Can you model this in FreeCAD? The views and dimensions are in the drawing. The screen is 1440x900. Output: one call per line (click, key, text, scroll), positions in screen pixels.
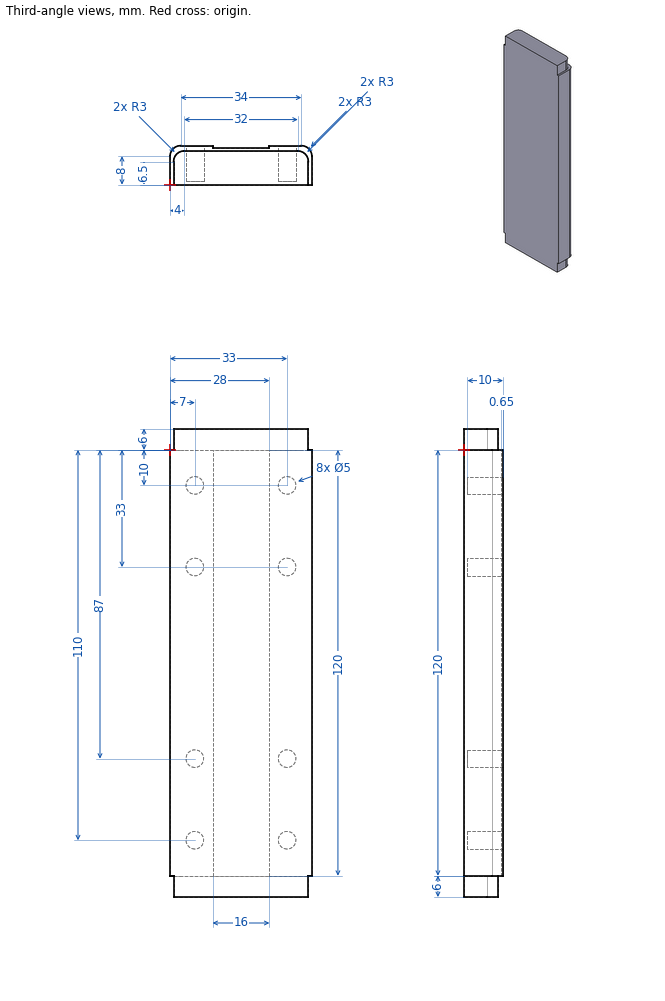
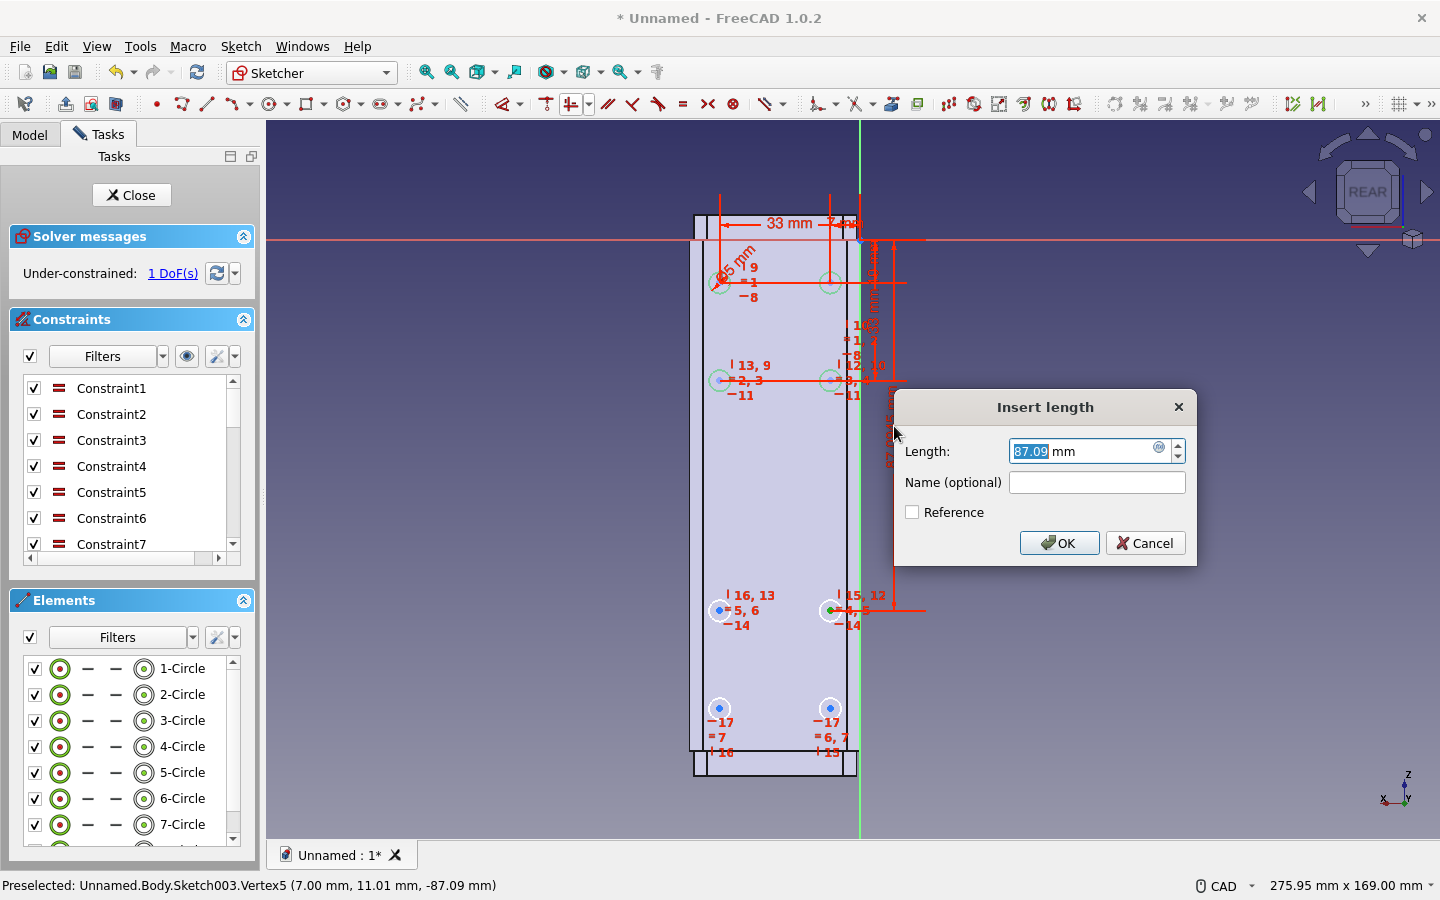
text(87)
key(Return)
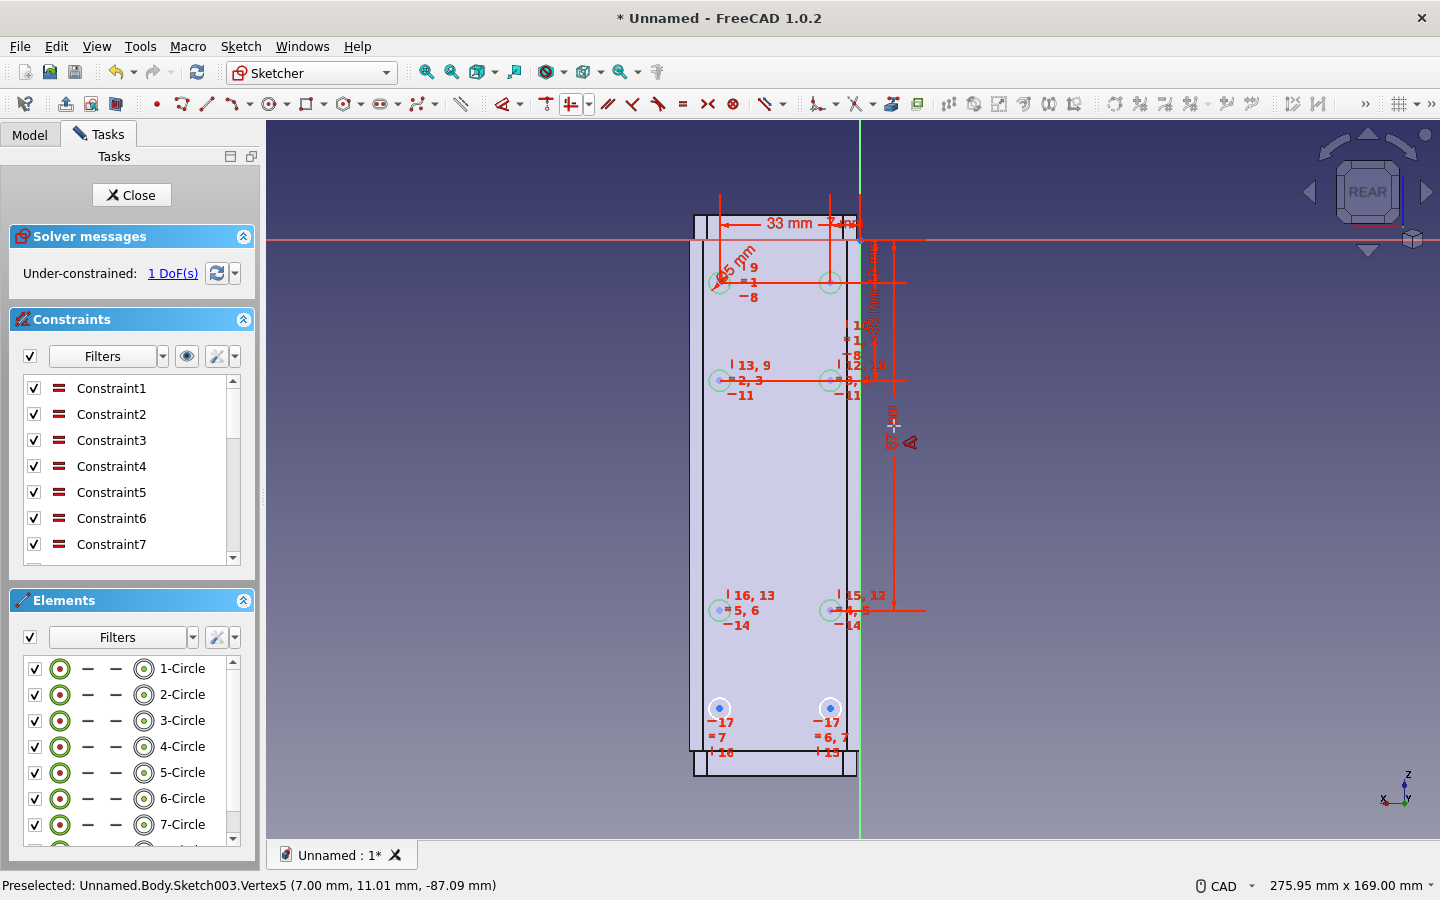
click(830, 709)
click(894, 475)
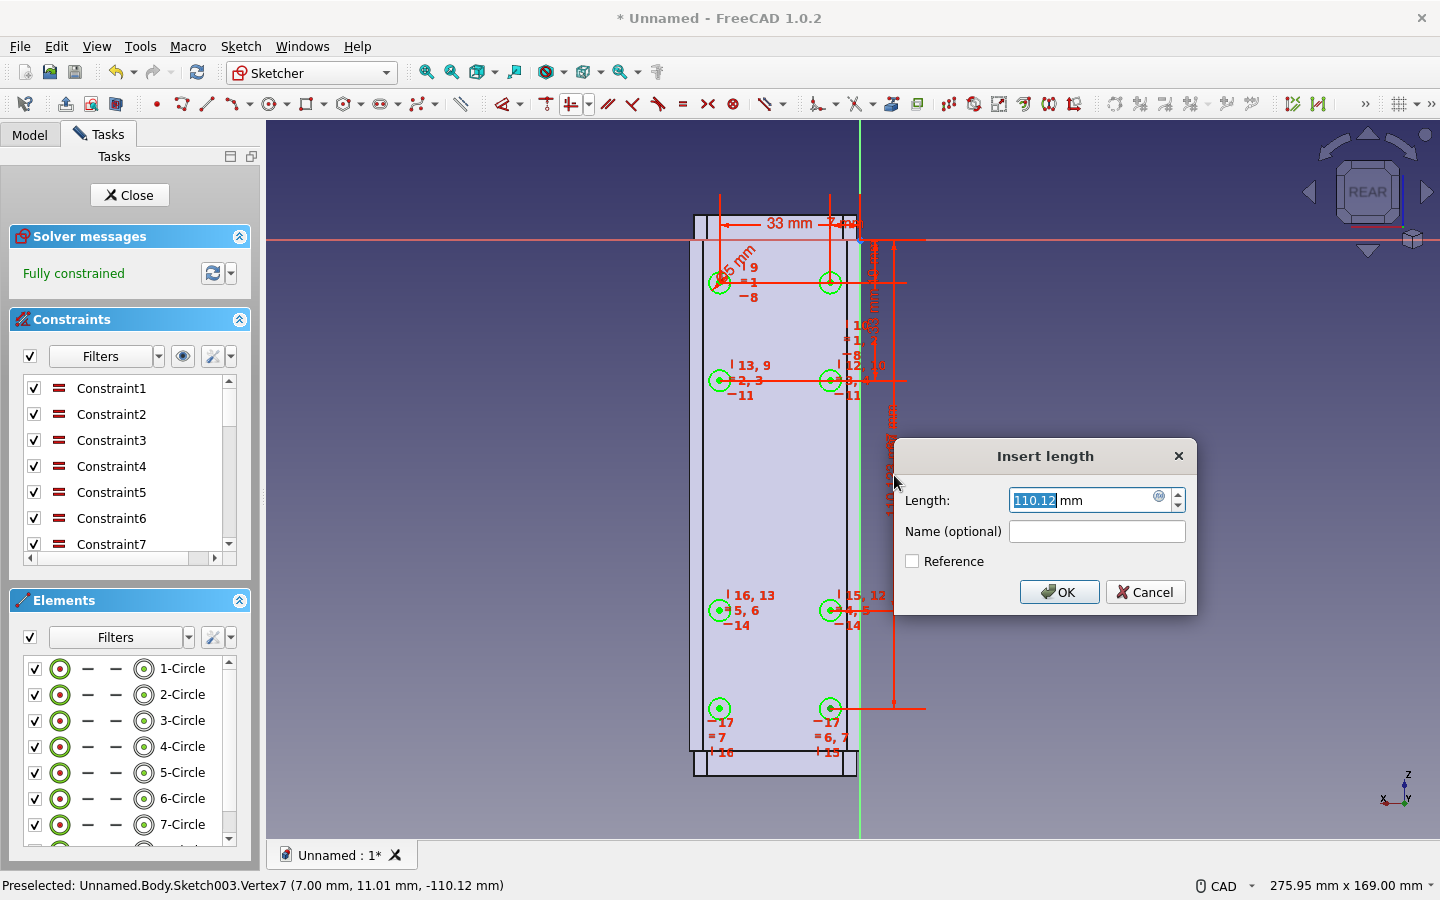
text(110)
key(Return)
key(Escape)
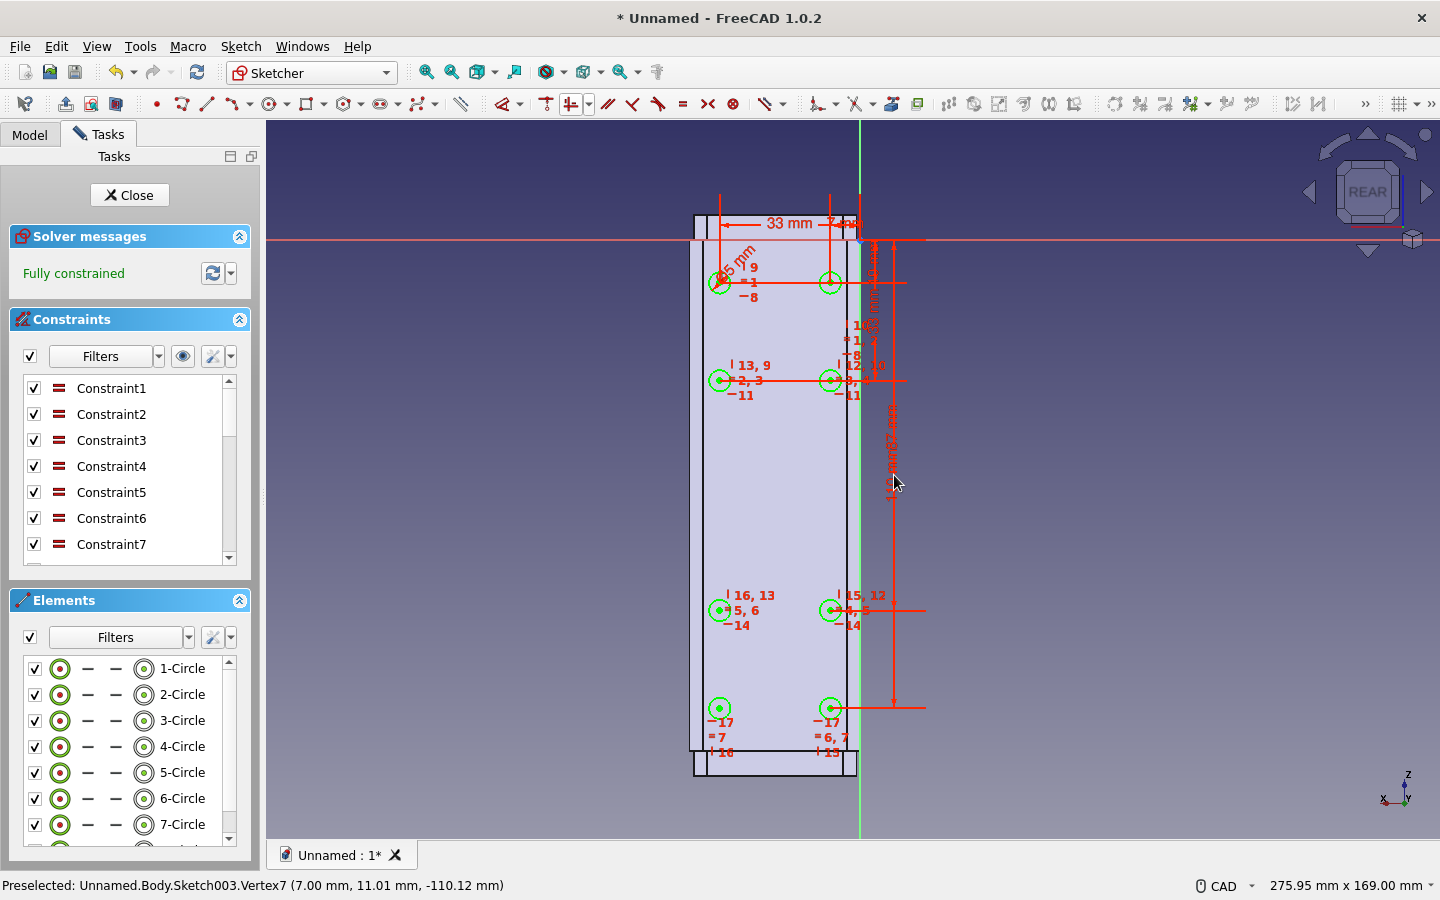
click(130, 195)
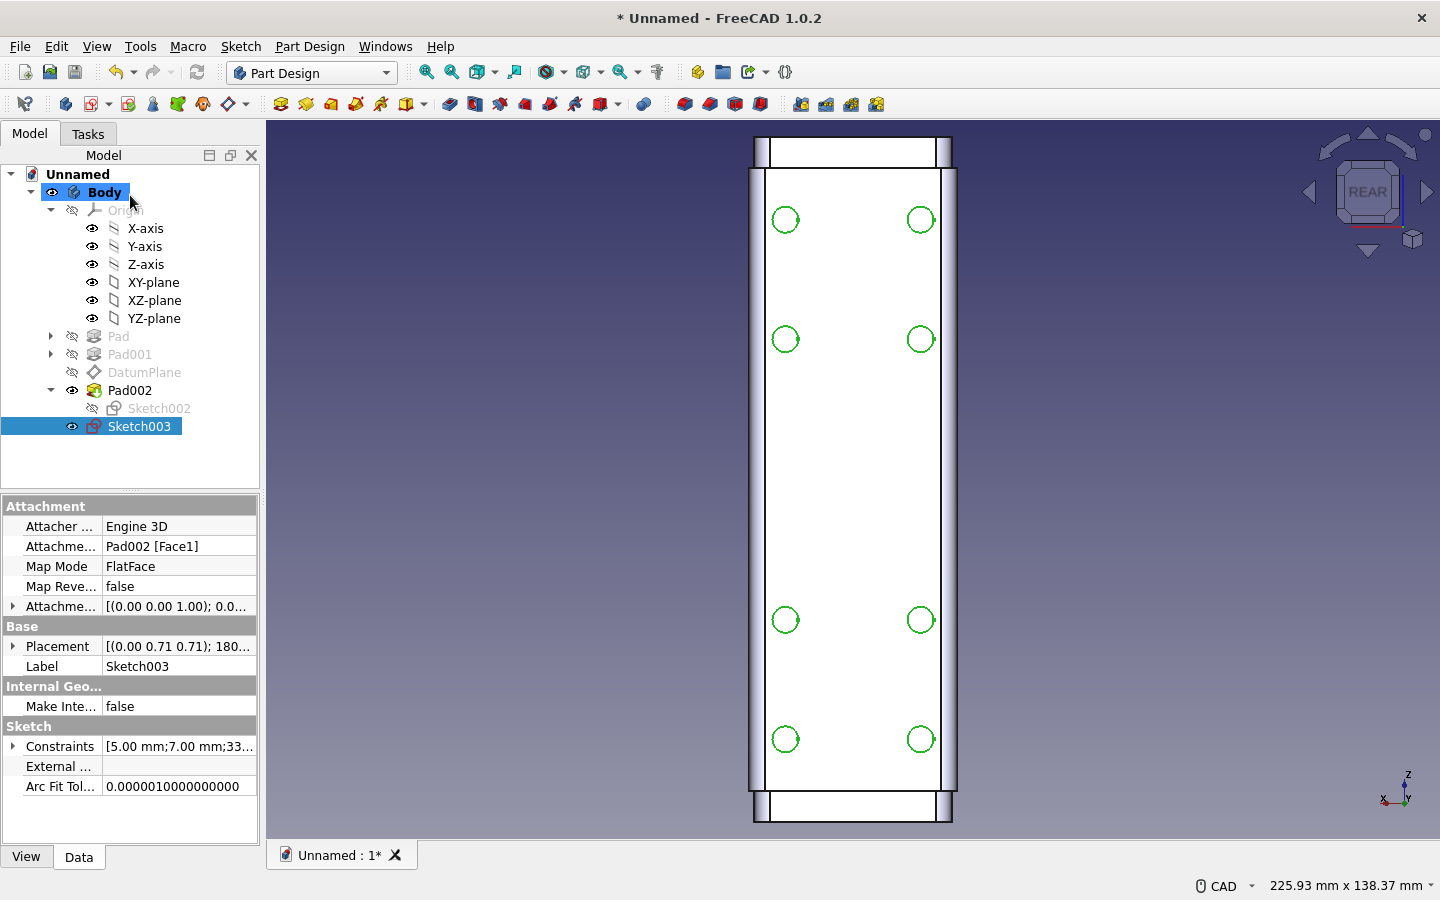
click(450, 104)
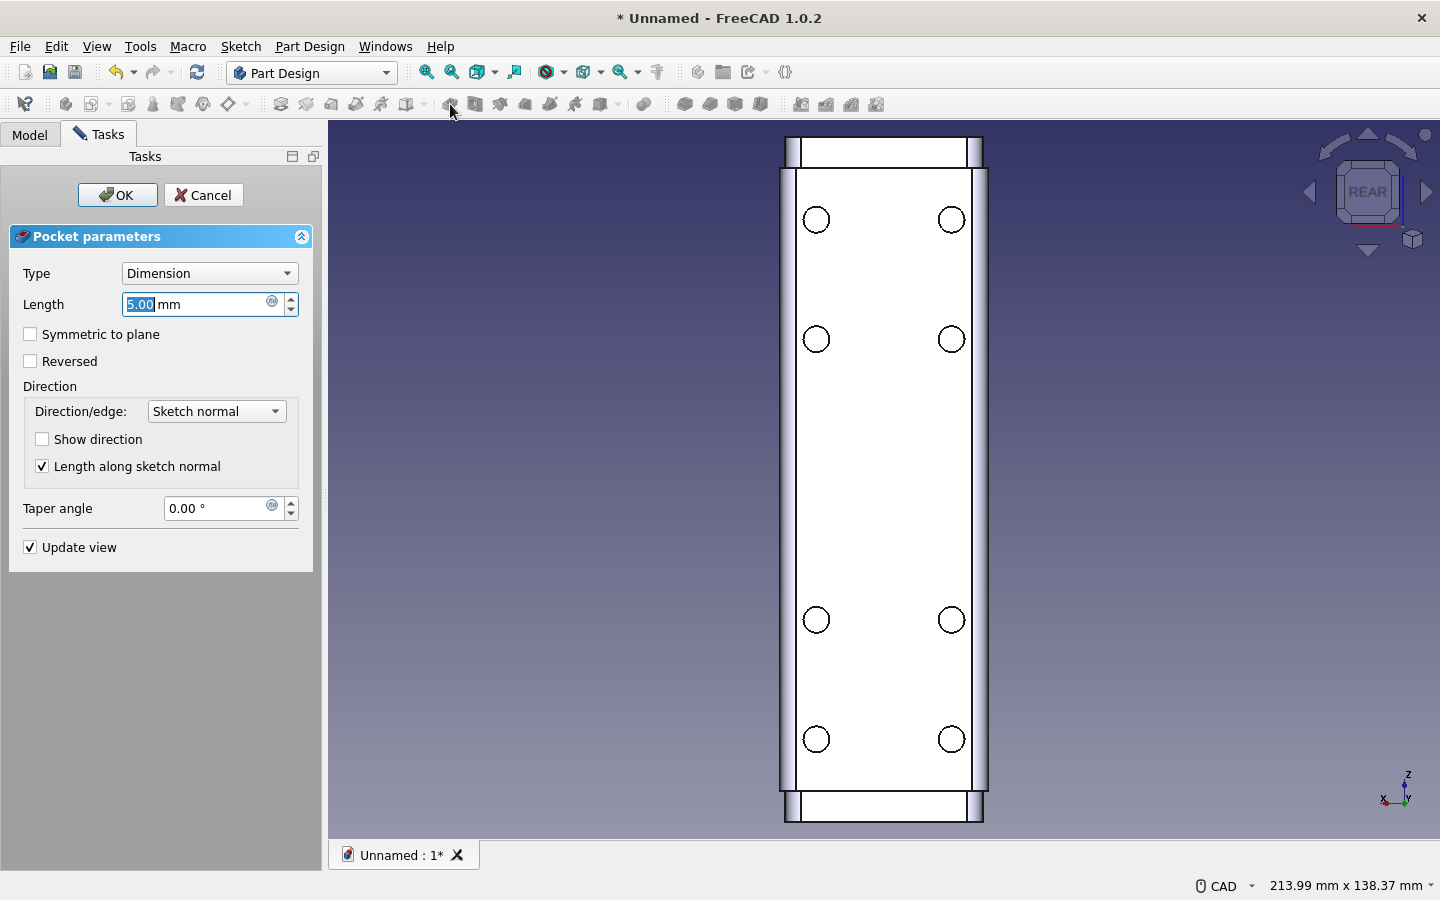
text(10)
key(Tab)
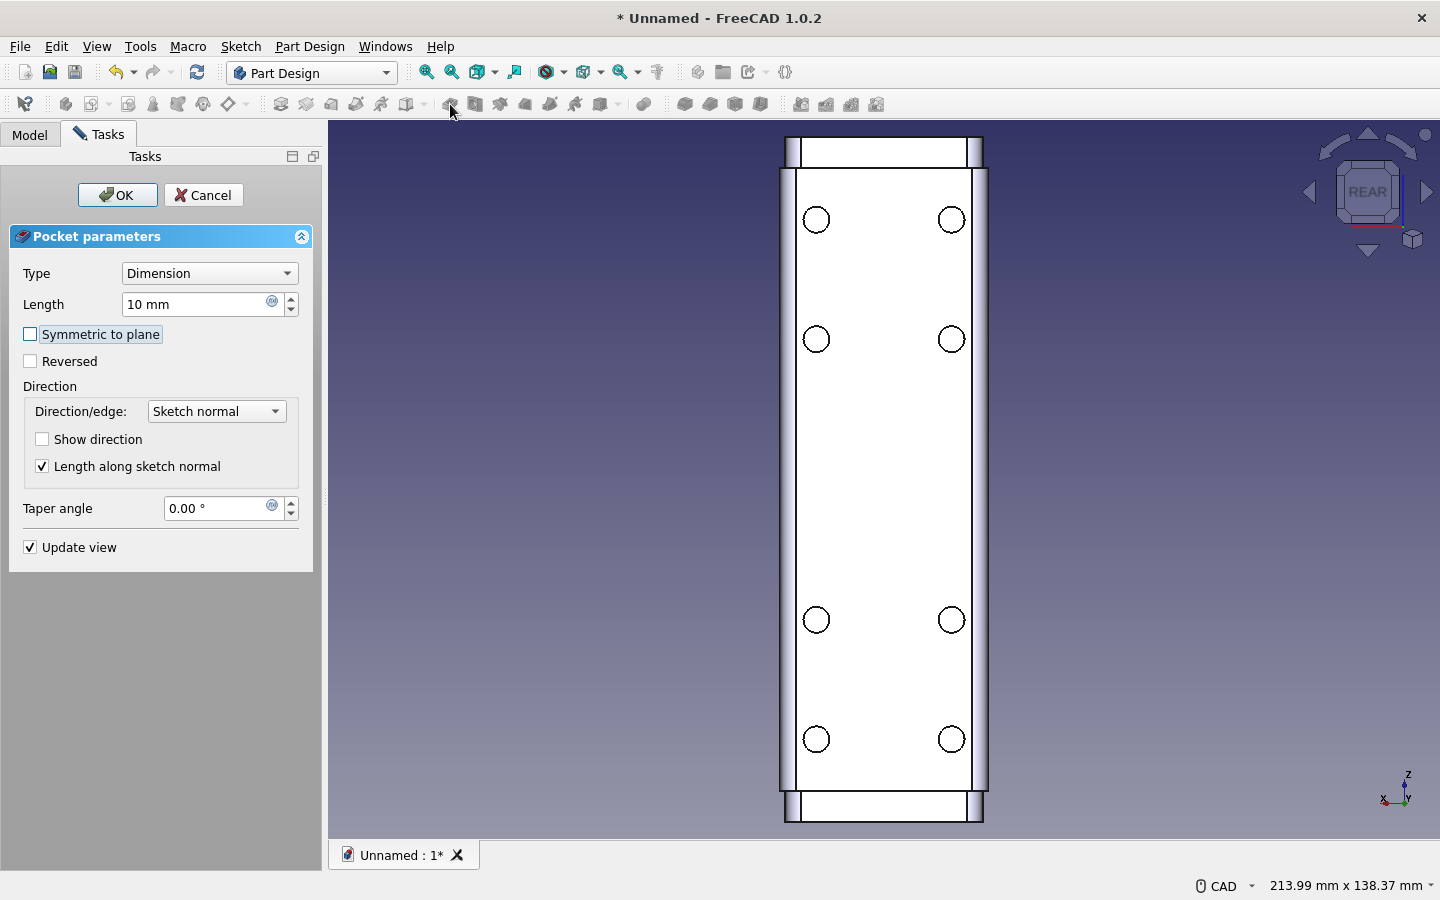
click(118, 195)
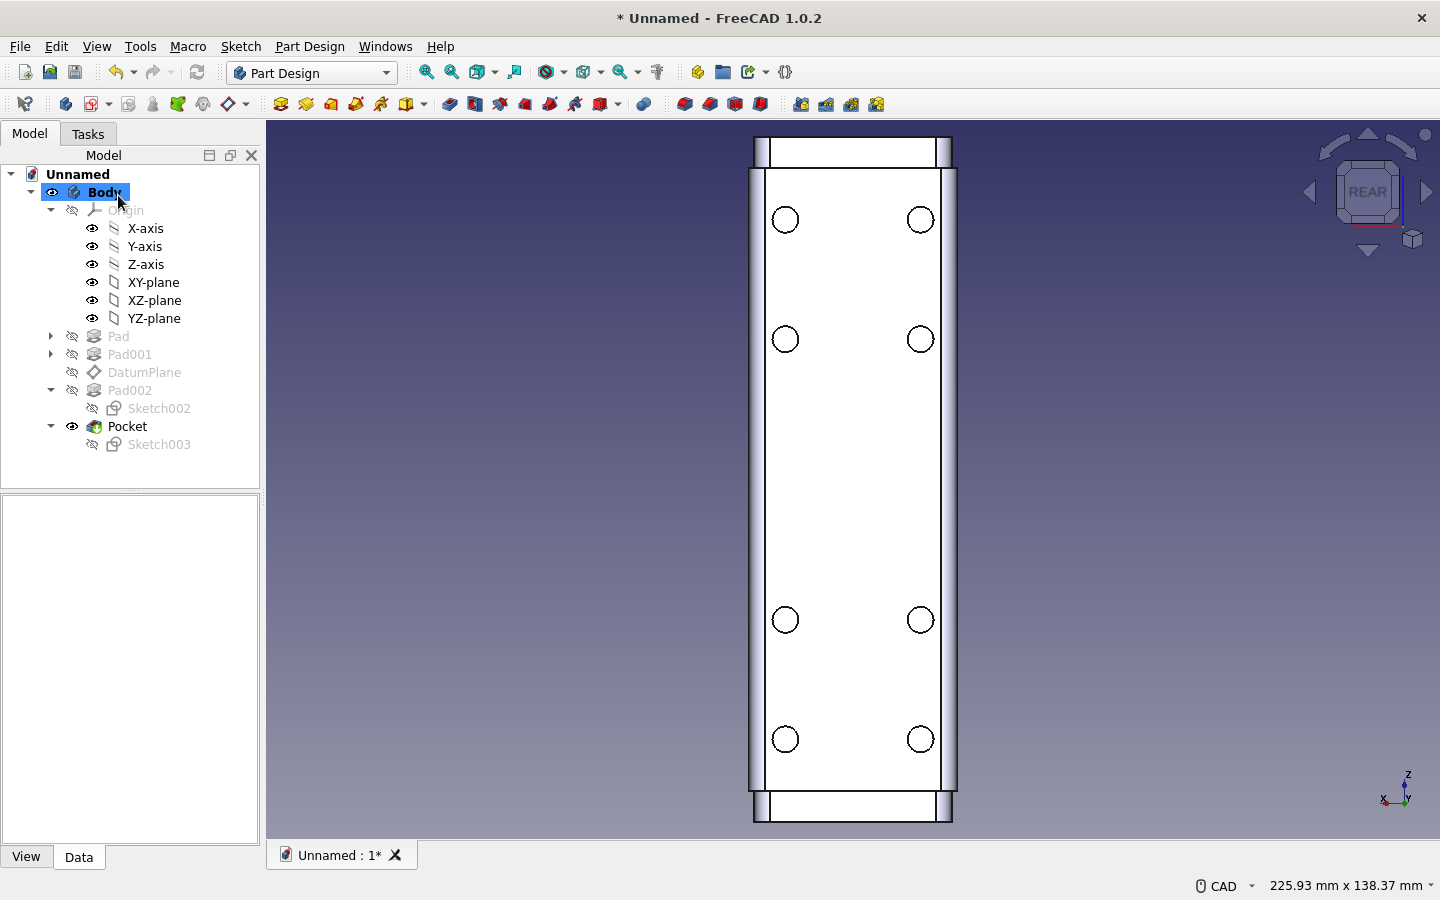
click(853, 479)